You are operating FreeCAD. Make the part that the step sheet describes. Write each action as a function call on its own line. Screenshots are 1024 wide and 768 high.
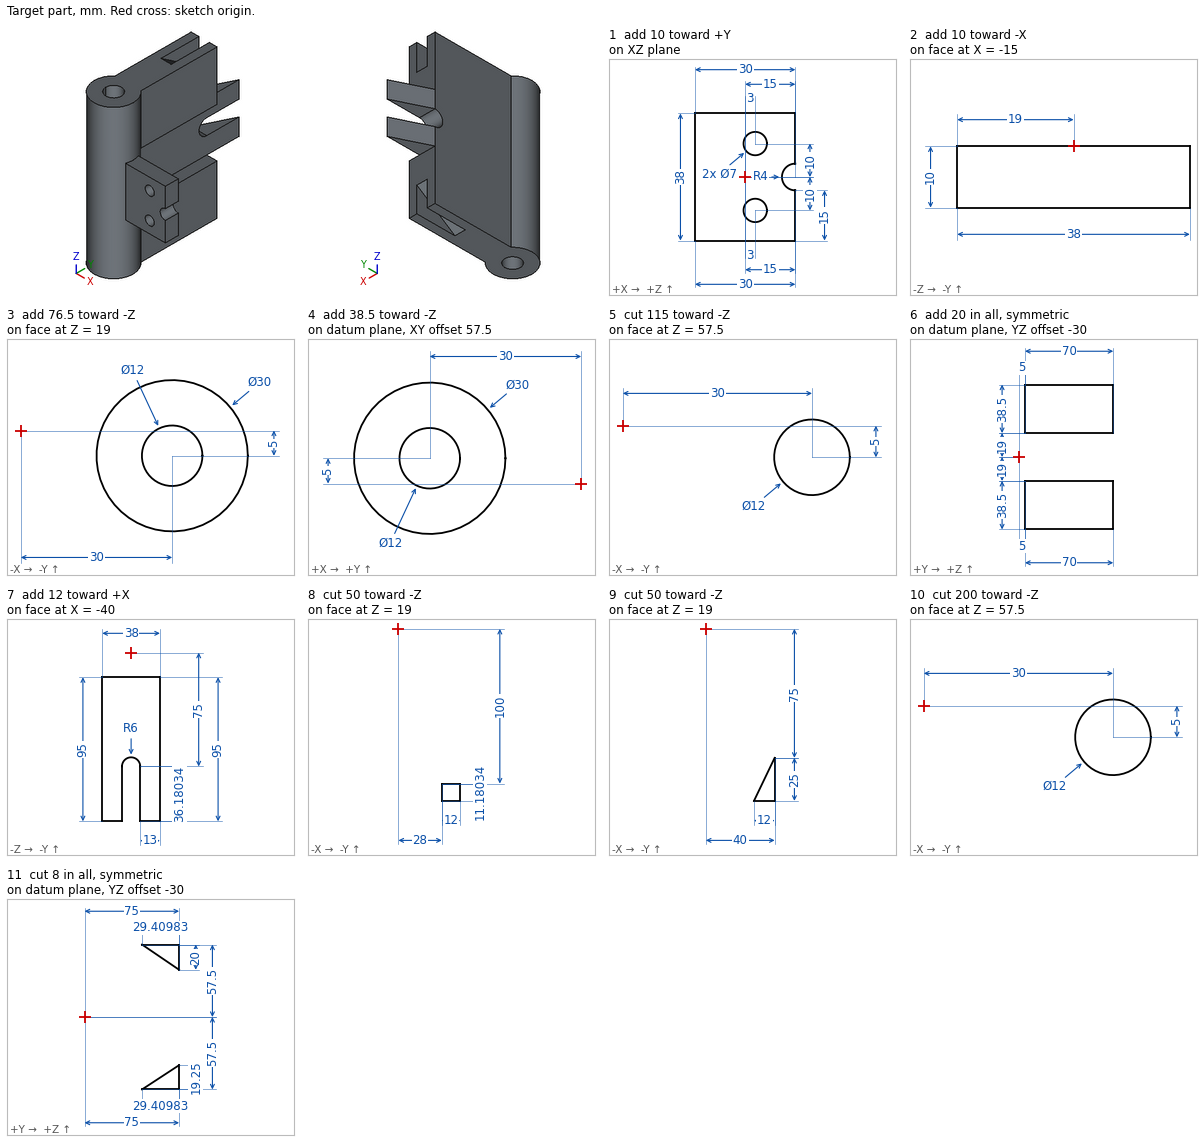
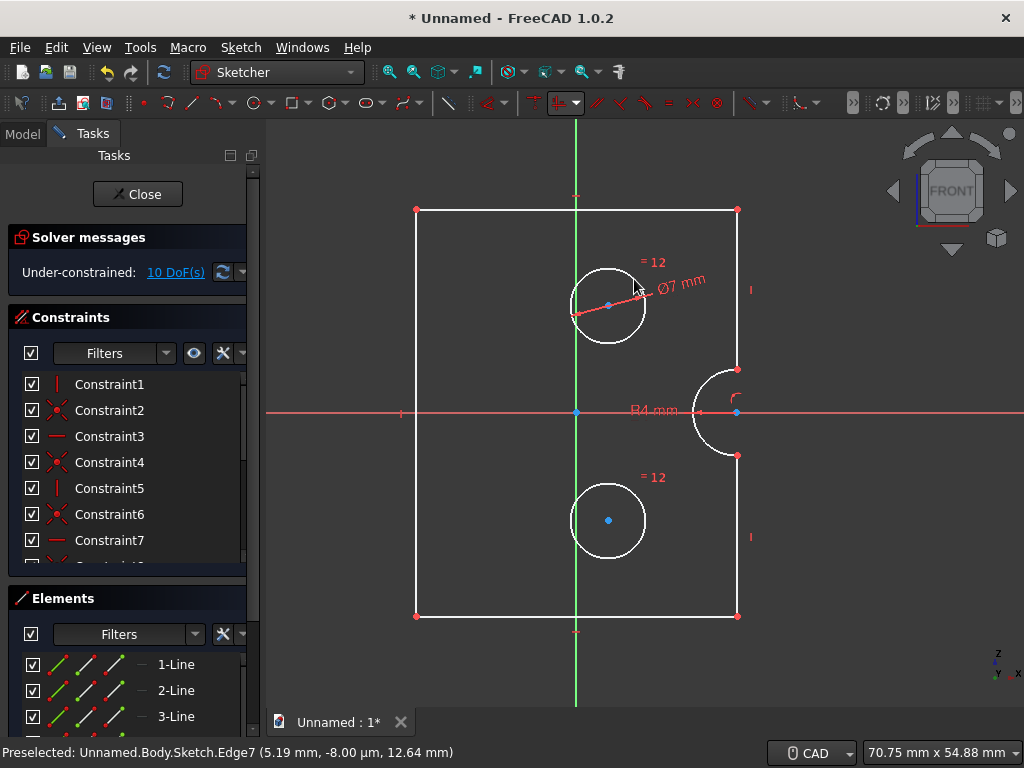
scroll(608, 306, up, 2)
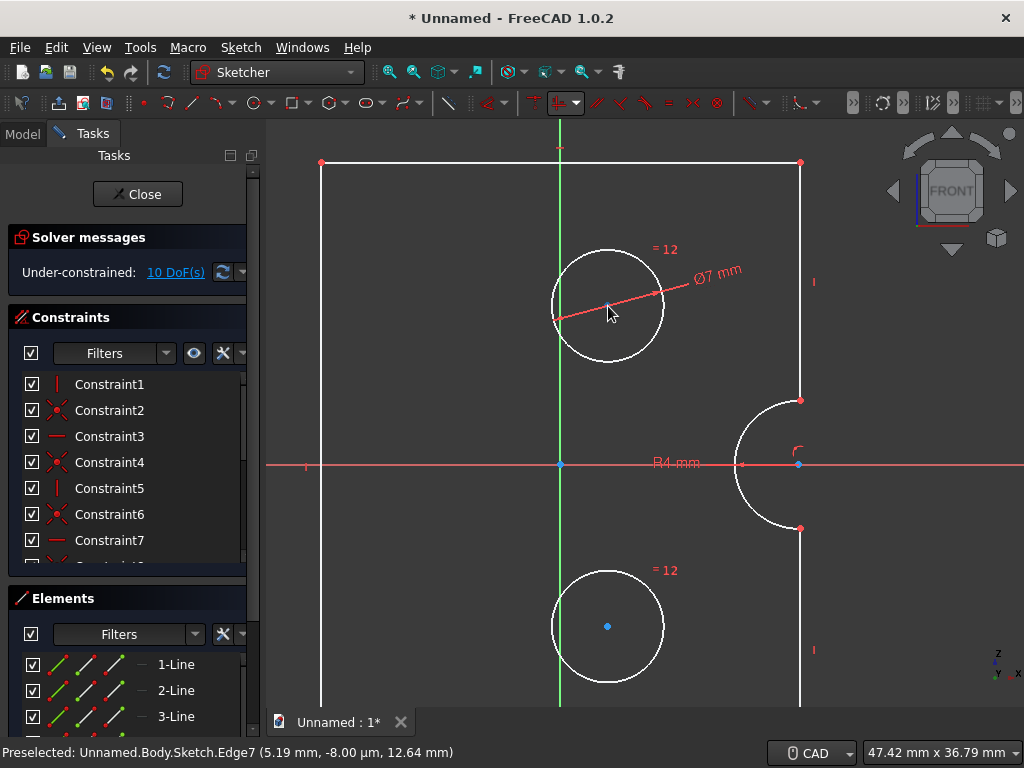
click(608, 306)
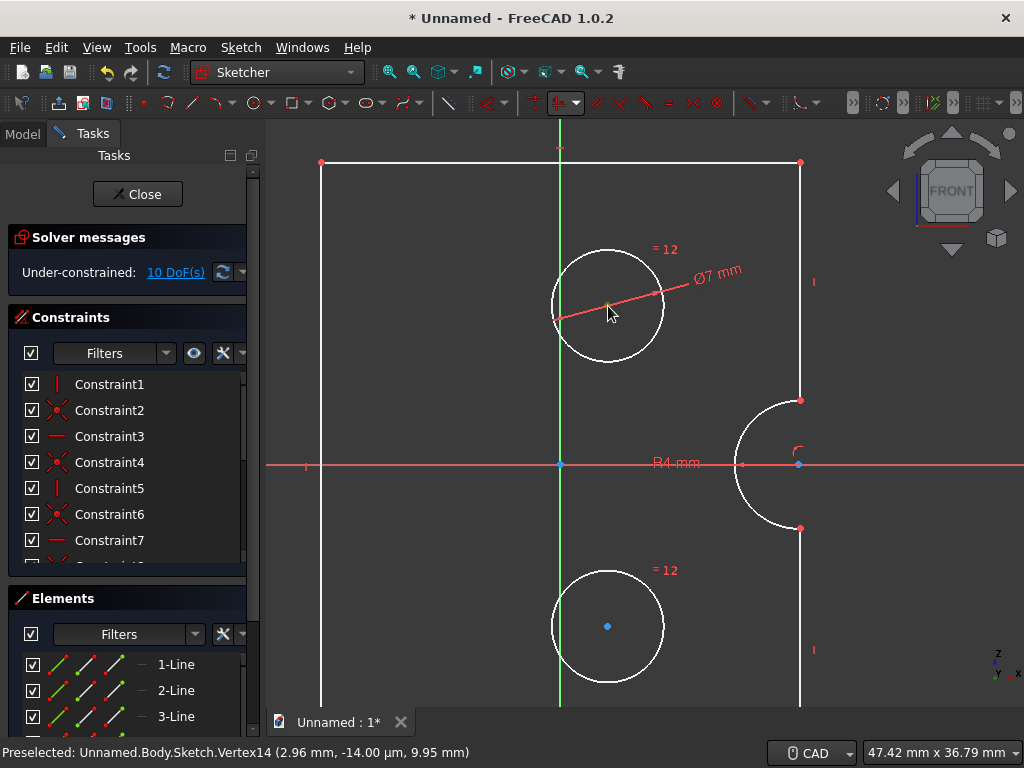
key(l)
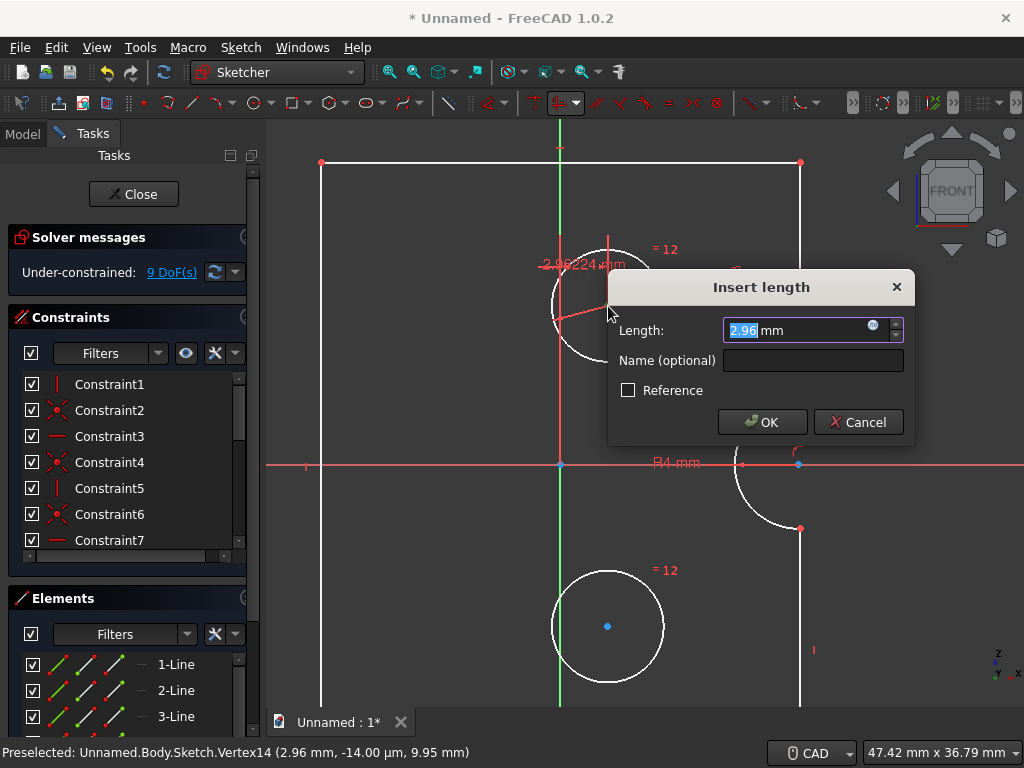
text(3)
key(Return)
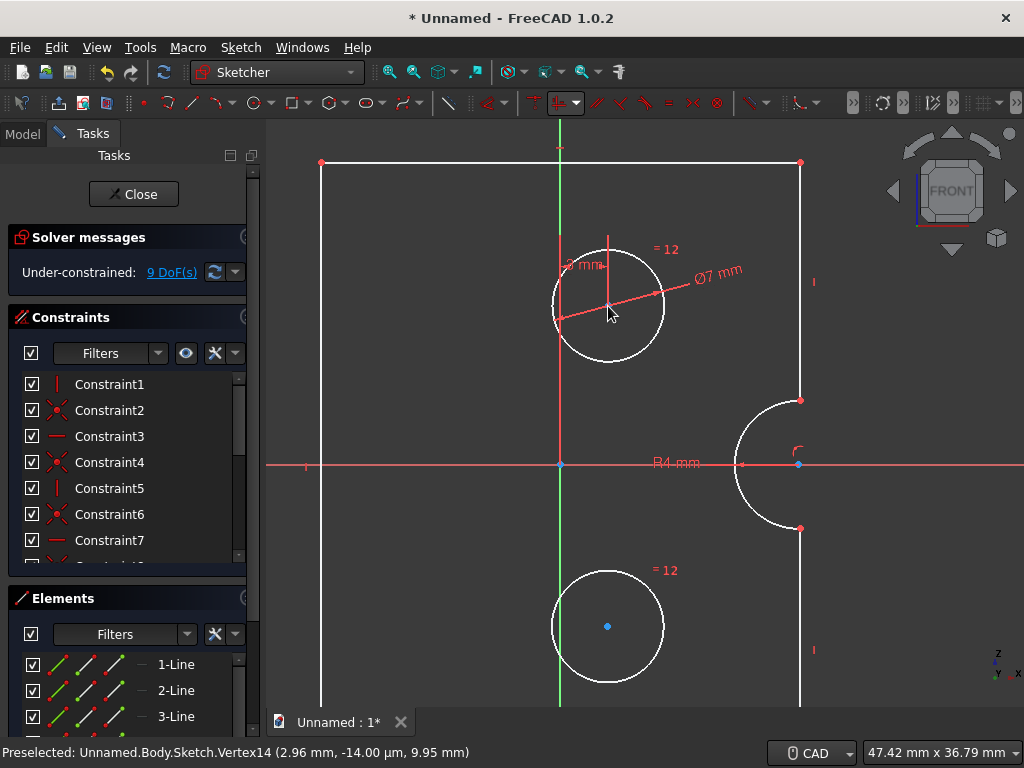
click(608, 627)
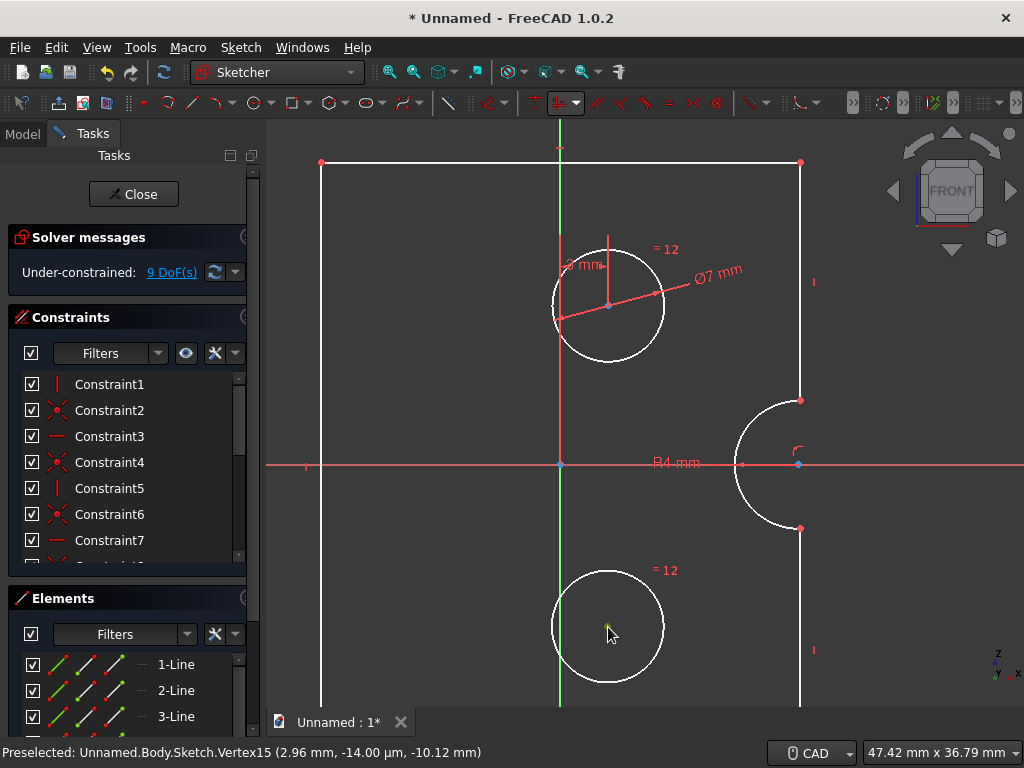
key(l)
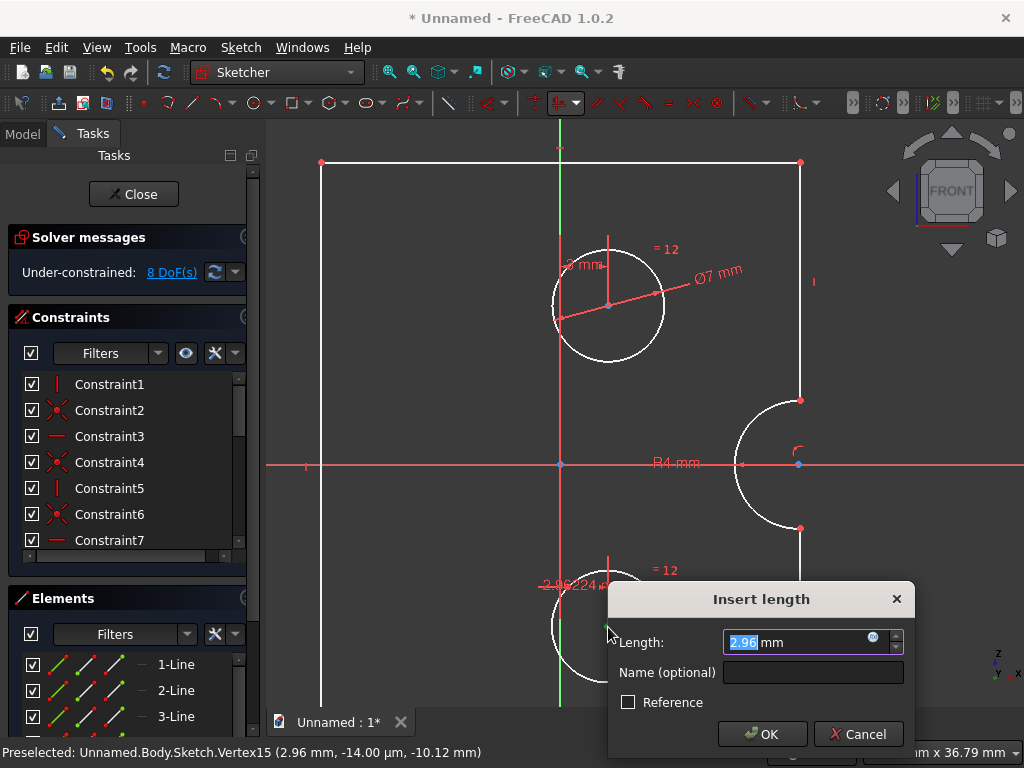
text(3)
key(Return)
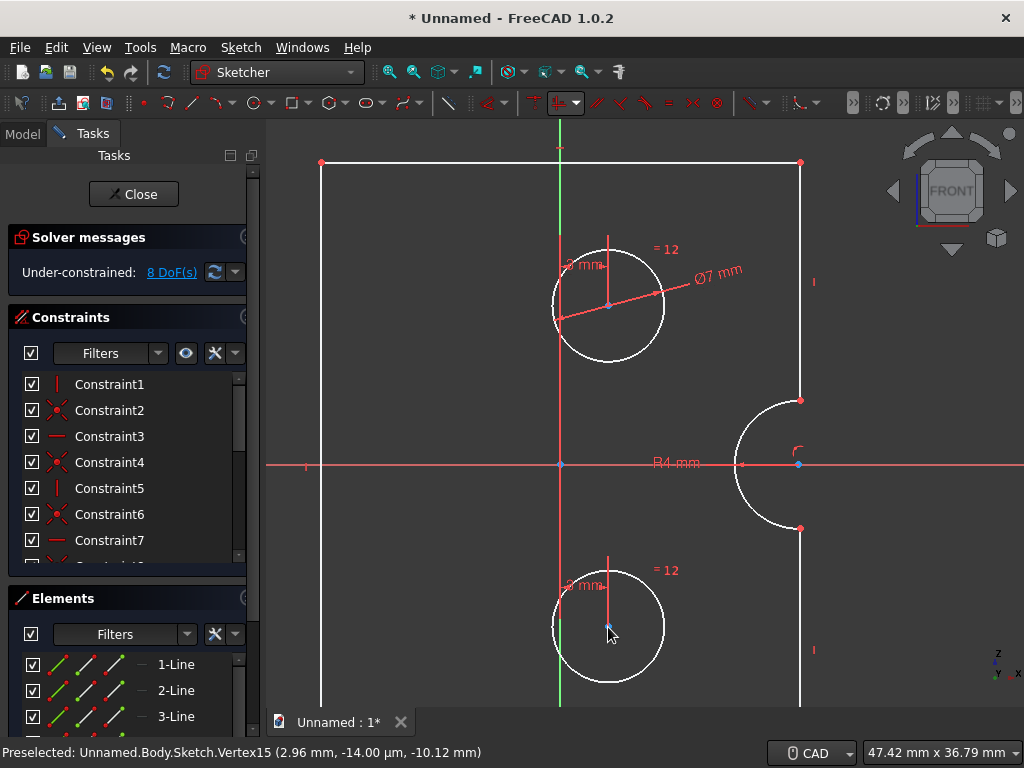
click(800, 601)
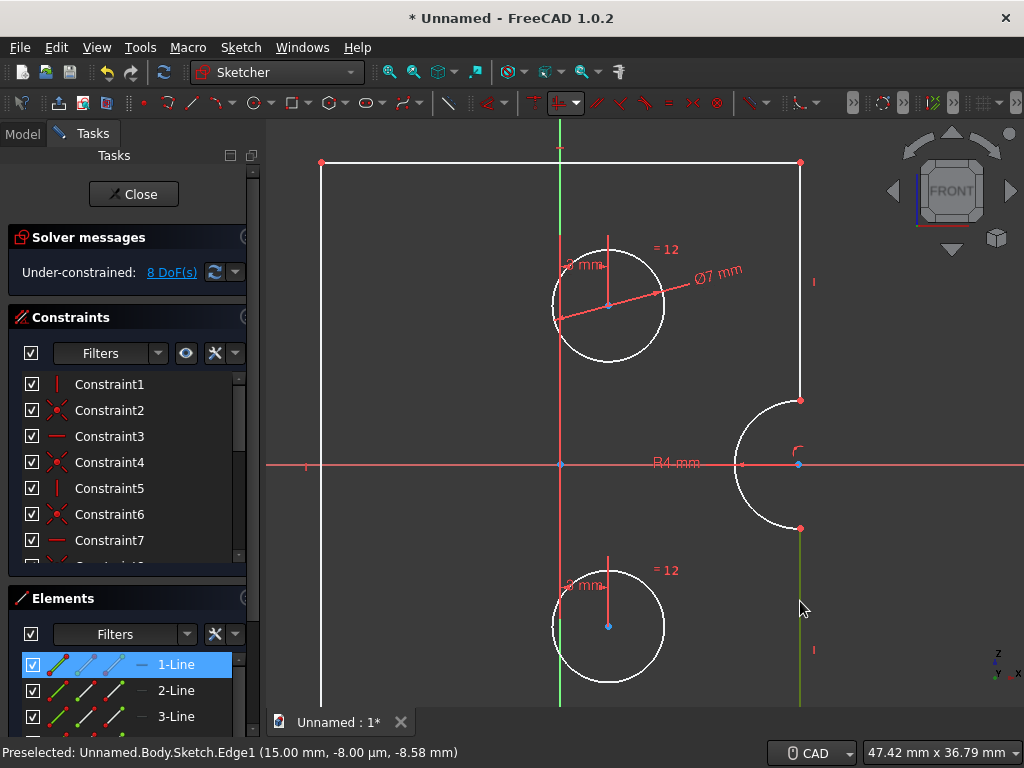
key(i)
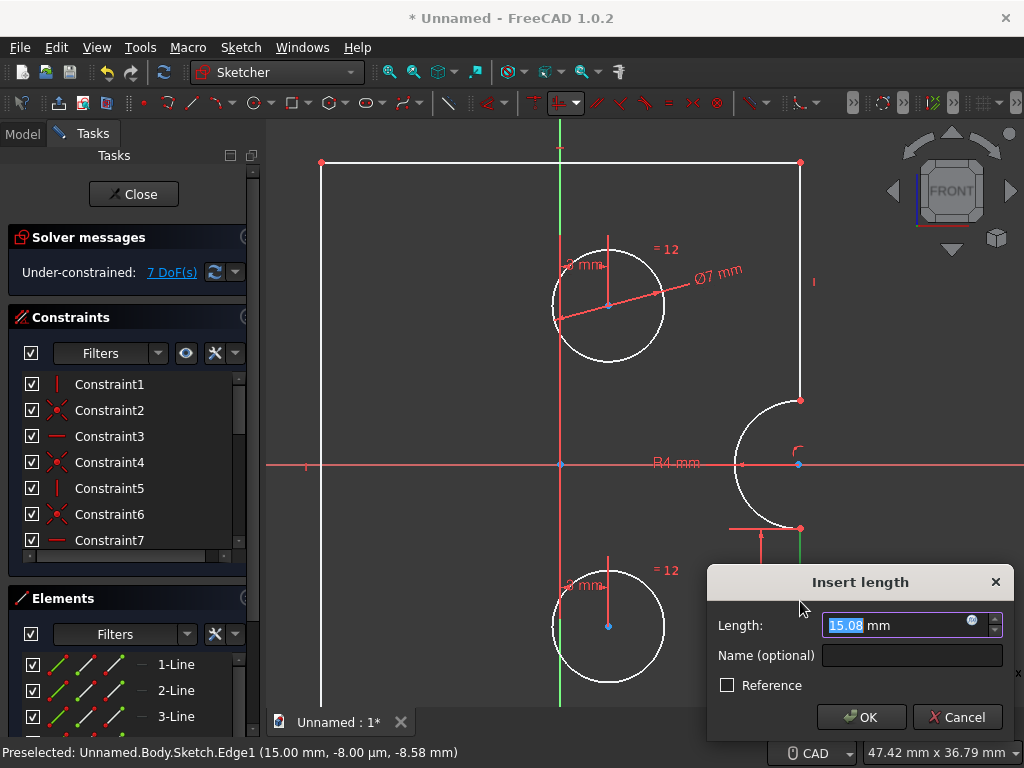
text(15)
key(Return)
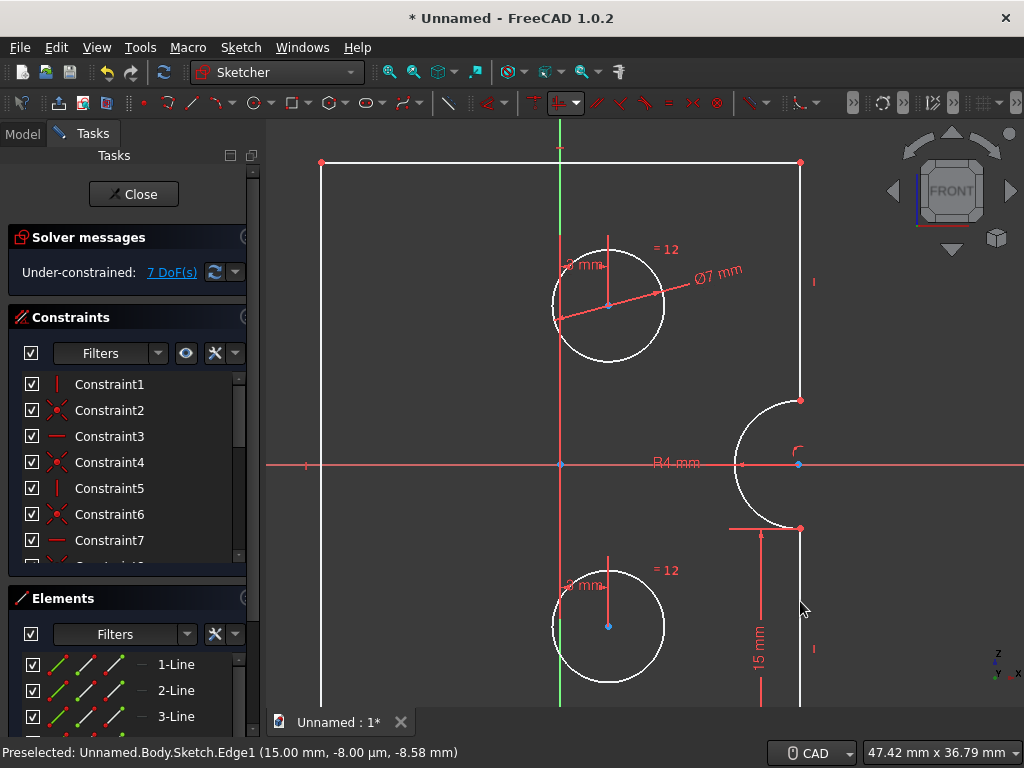
scroll(609, 308, down, 2)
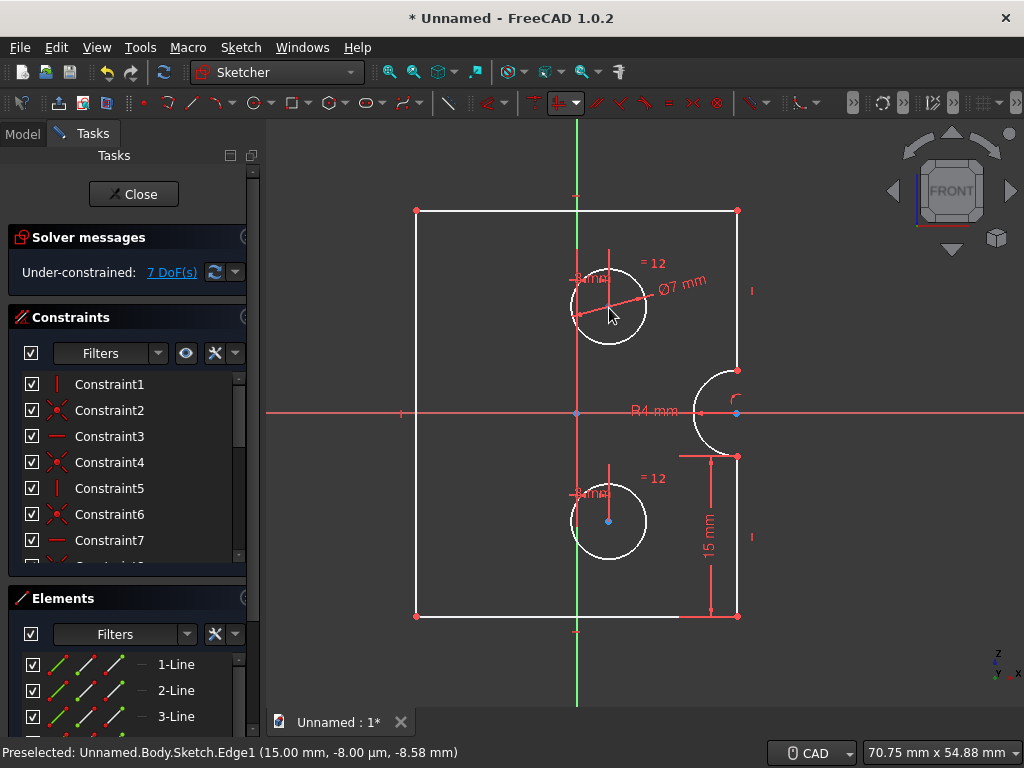
click(641, 617)